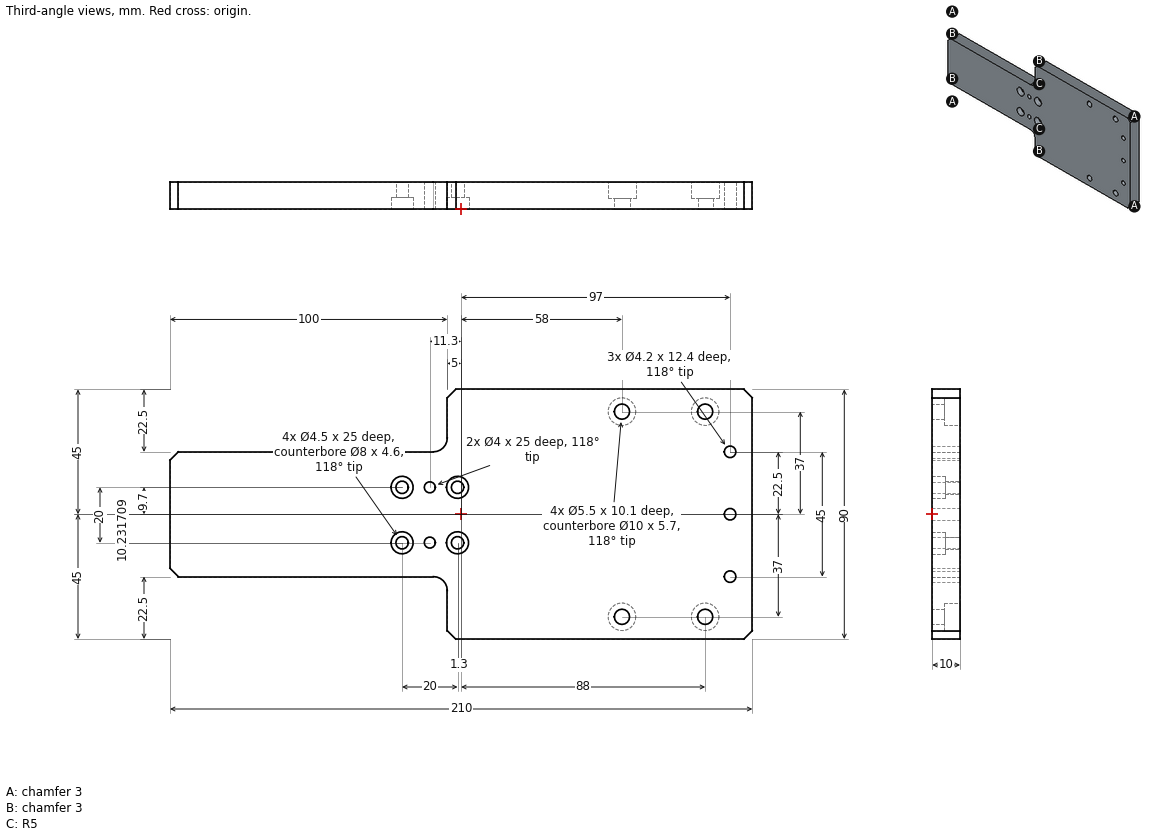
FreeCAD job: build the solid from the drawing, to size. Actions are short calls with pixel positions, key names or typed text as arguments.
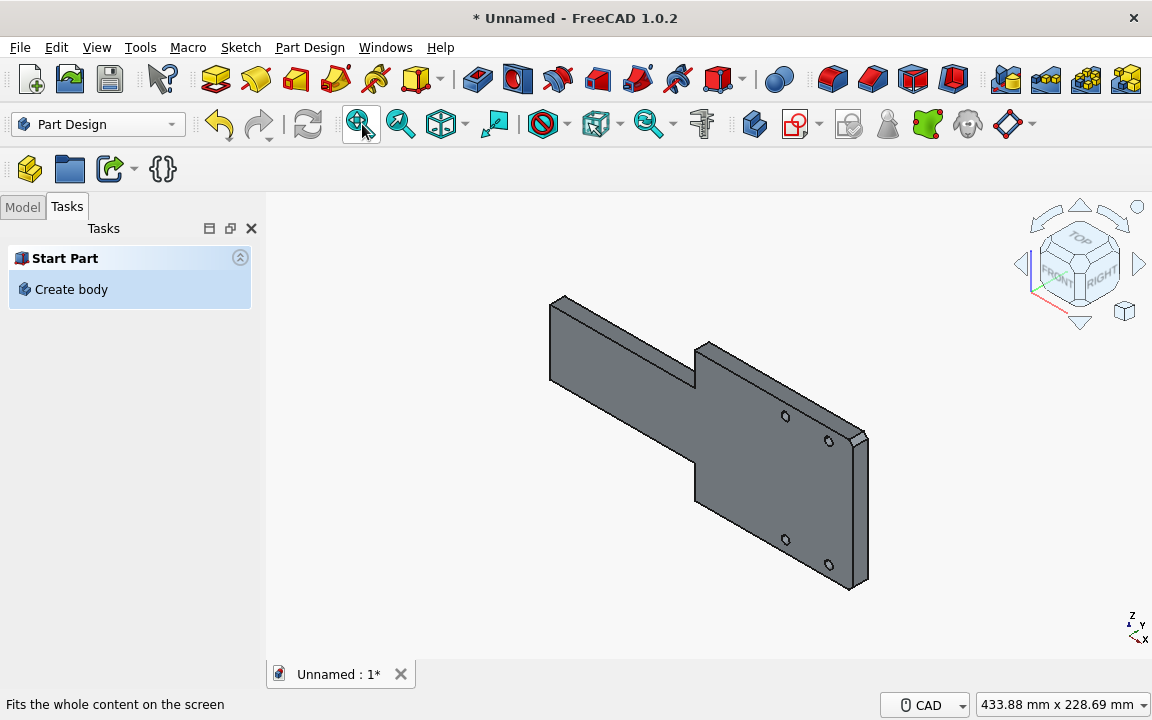
key(2)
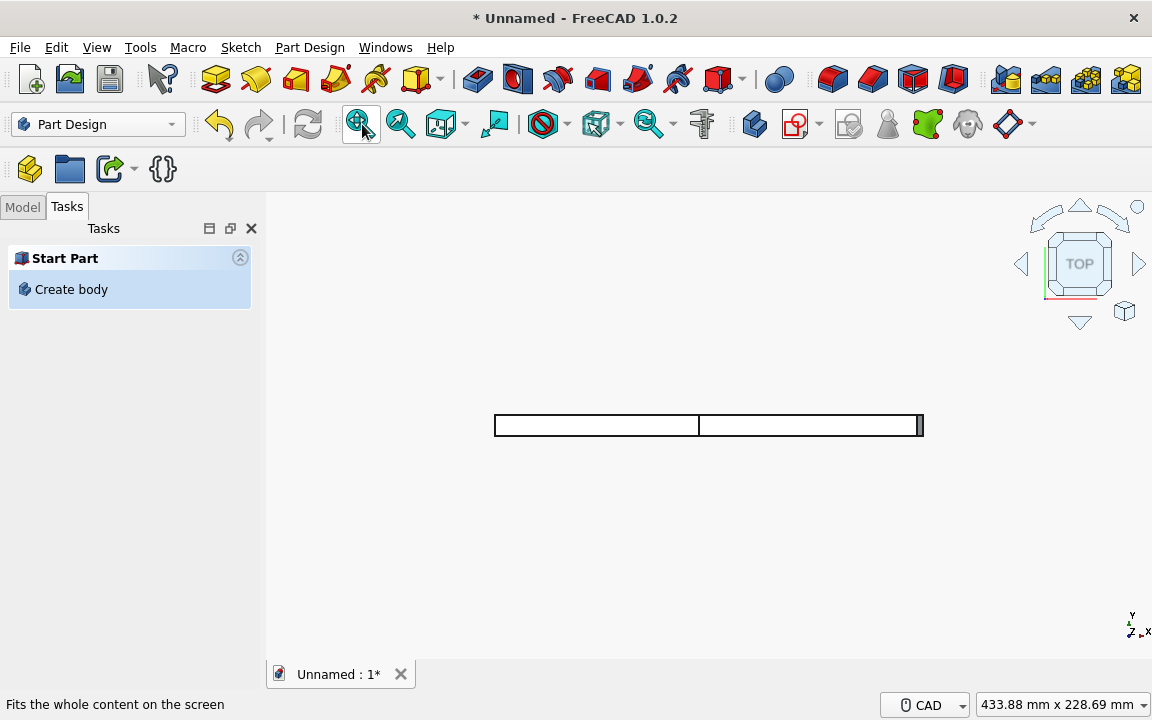
click(495, 424)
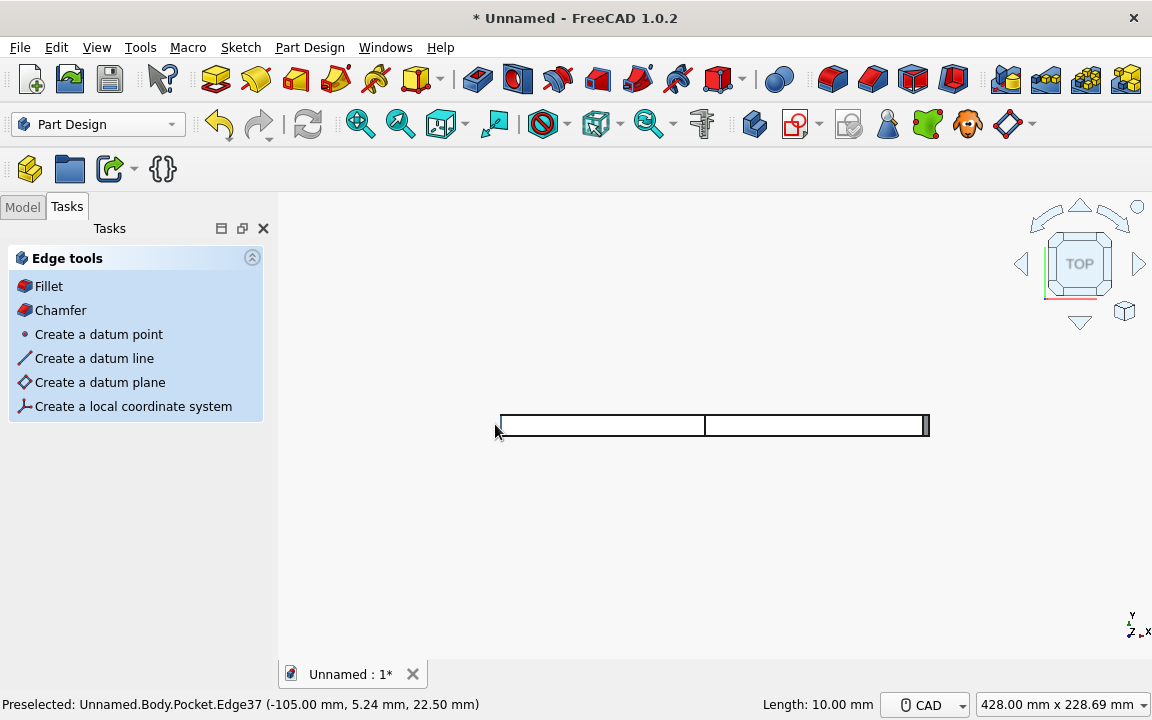
click(705, 424, ctrl)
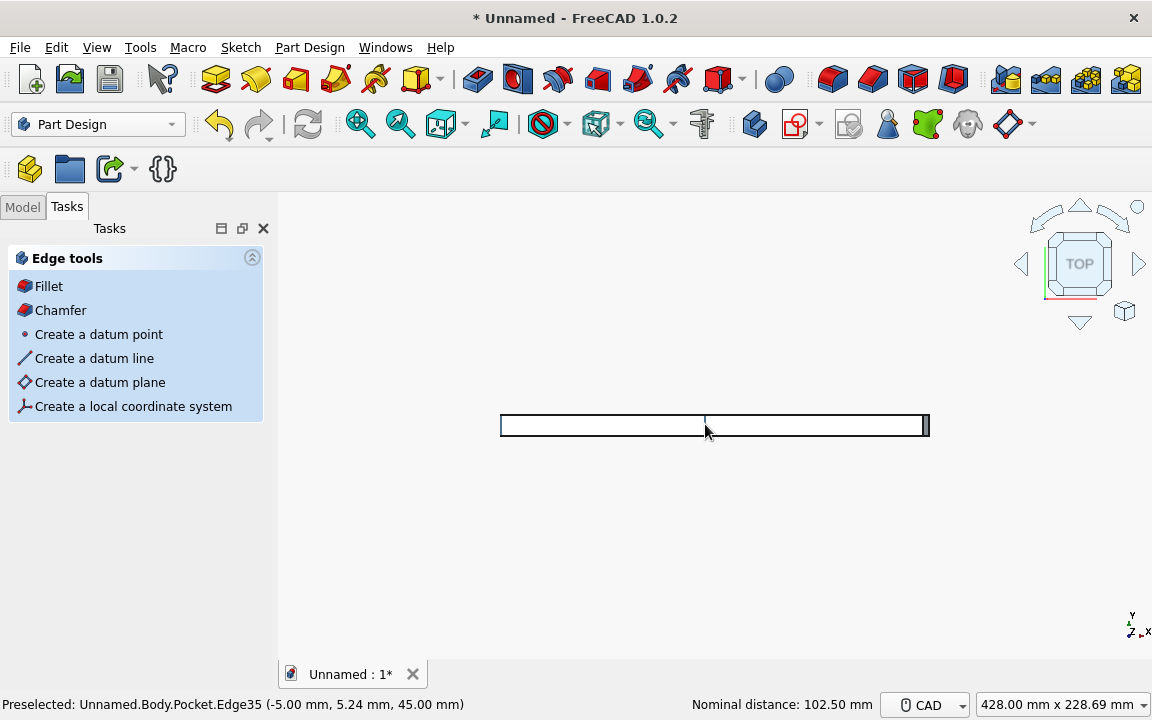
scroll(705, 424, up, 4)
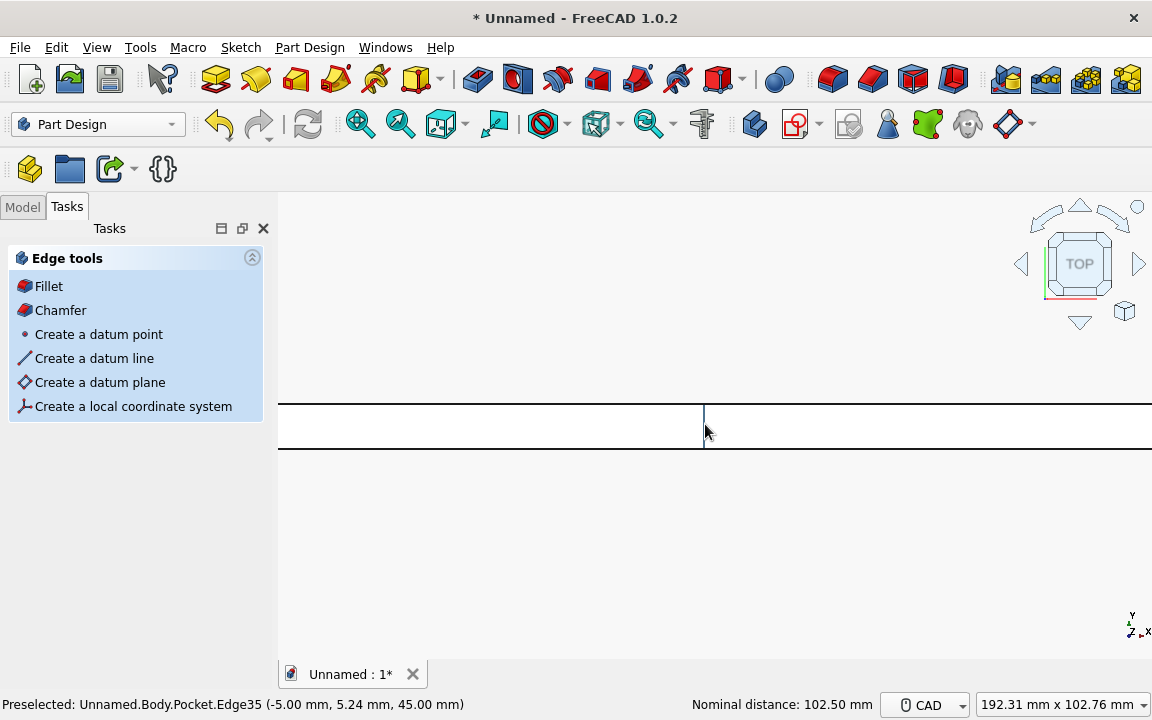
click(362, 124)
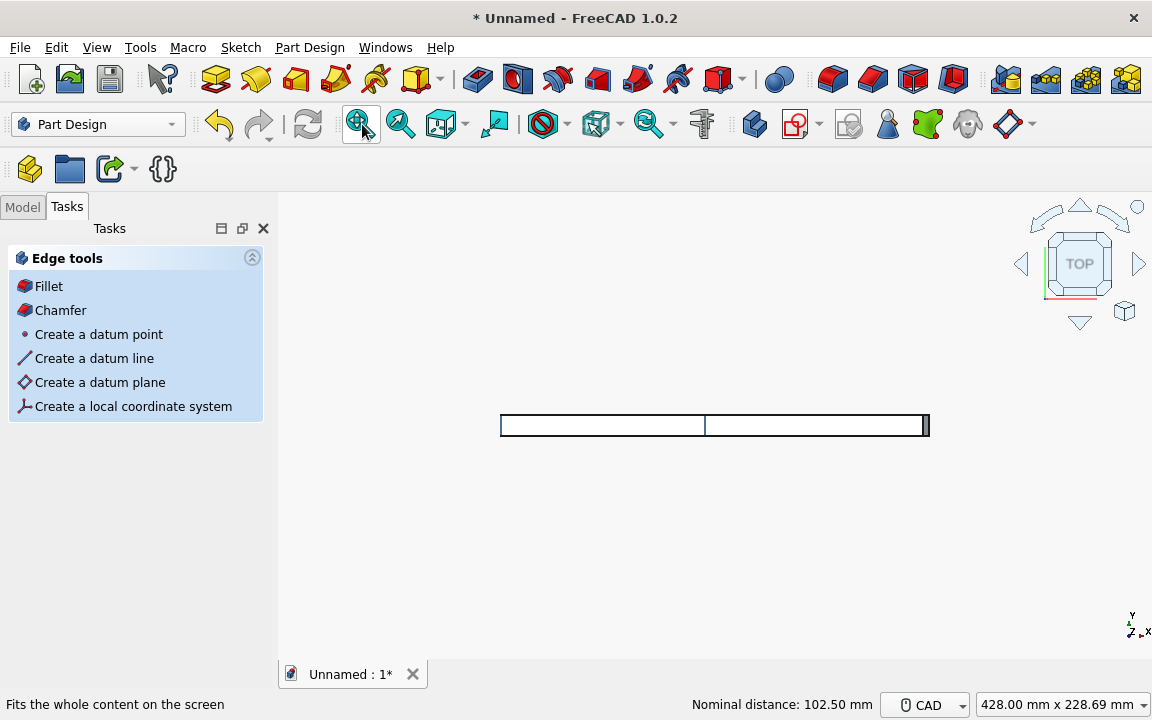
key(1)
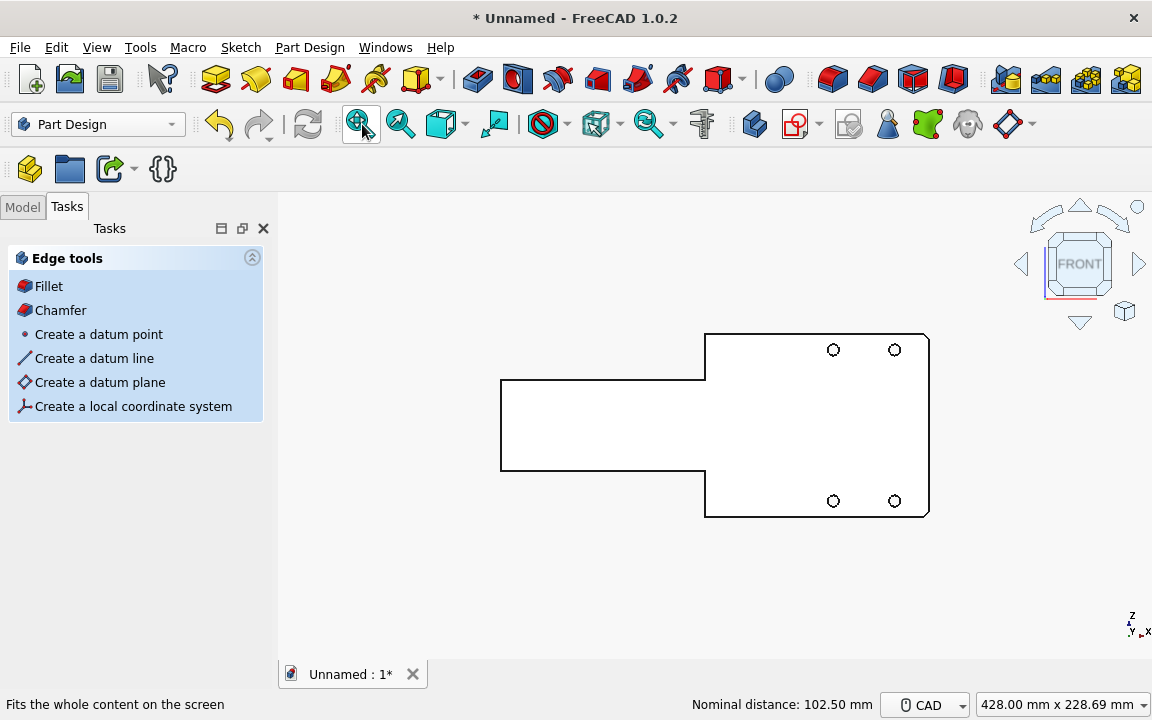
scroll(705, 516, up, 4)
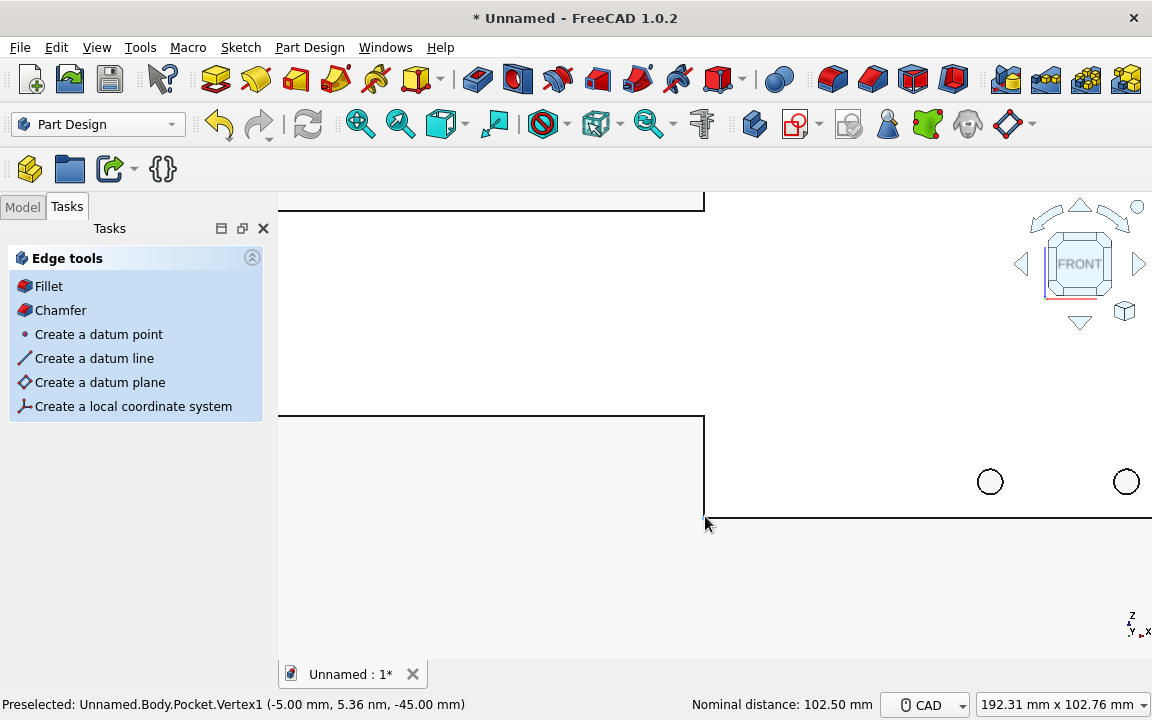
click(362, 124)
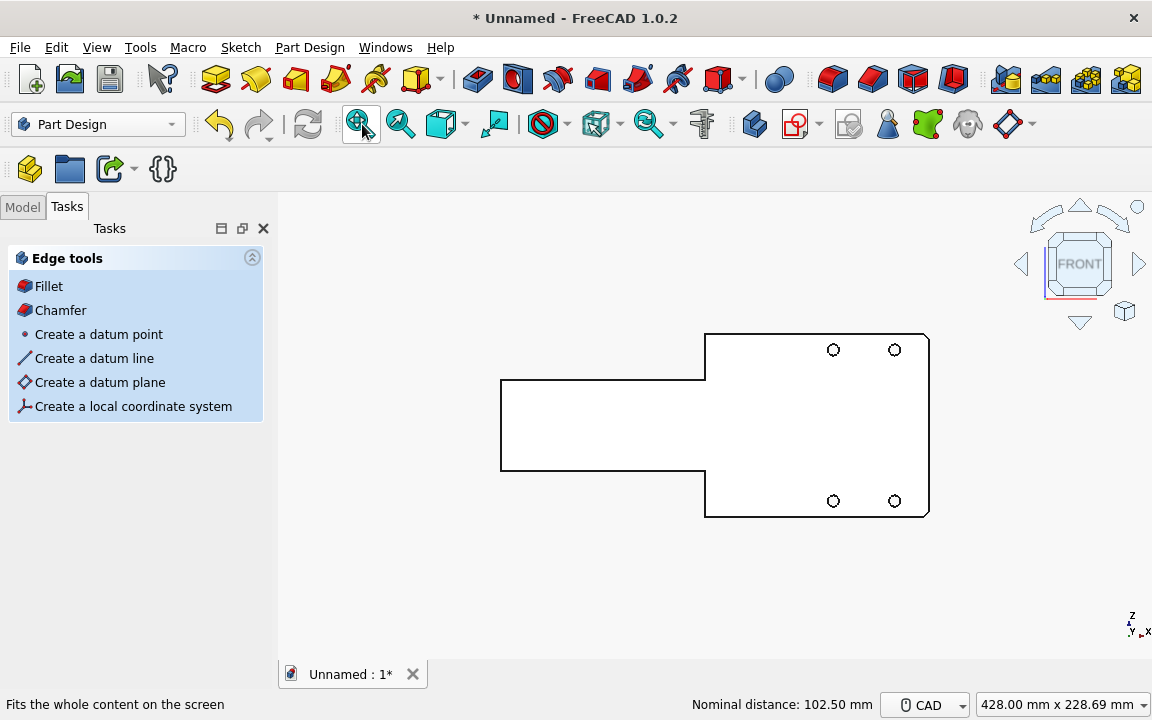
key(3)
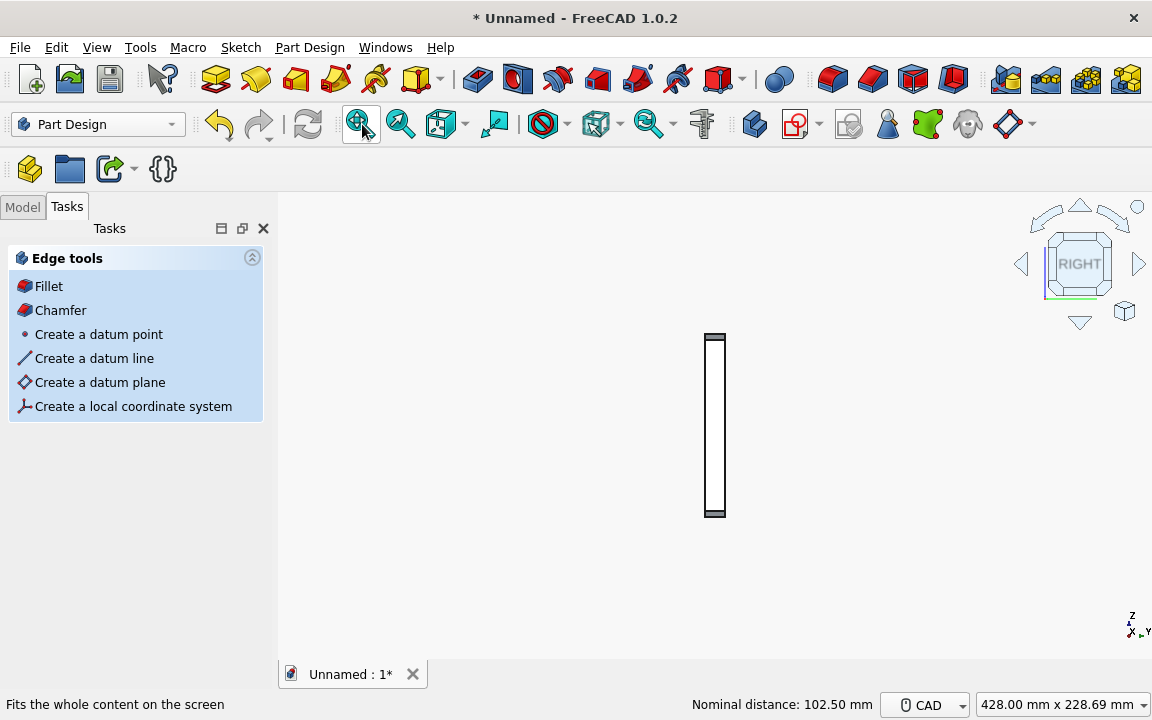
click(362, 124)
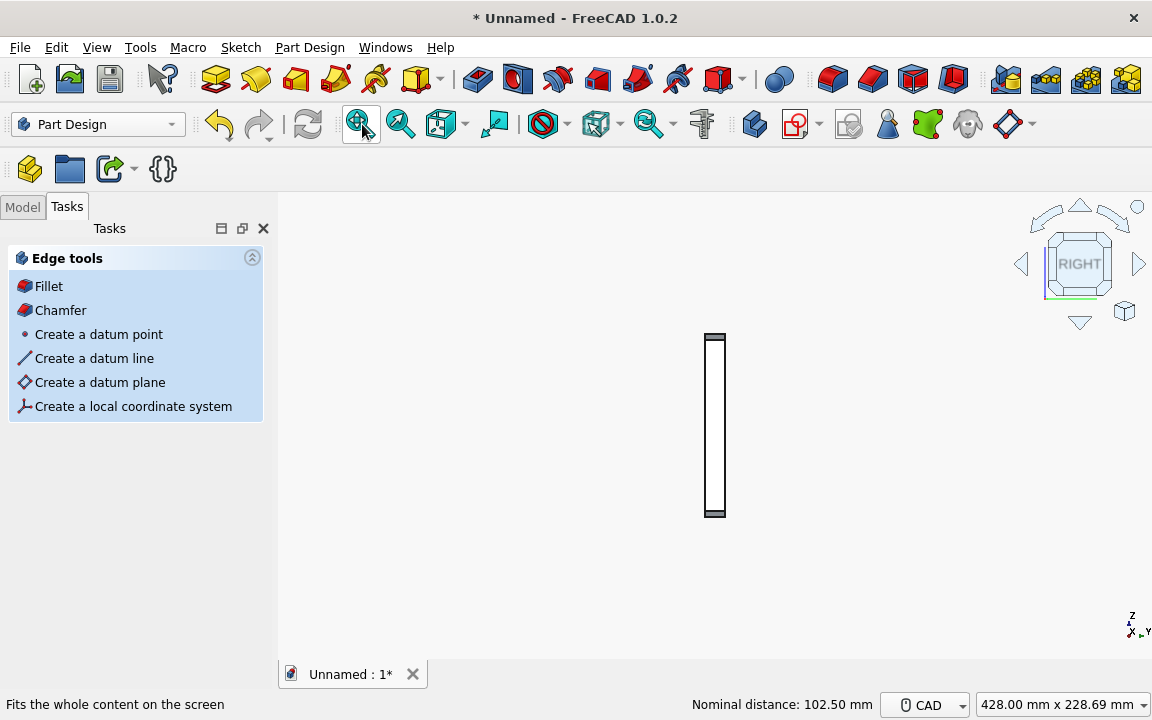
scroll(715, 516, up, 4)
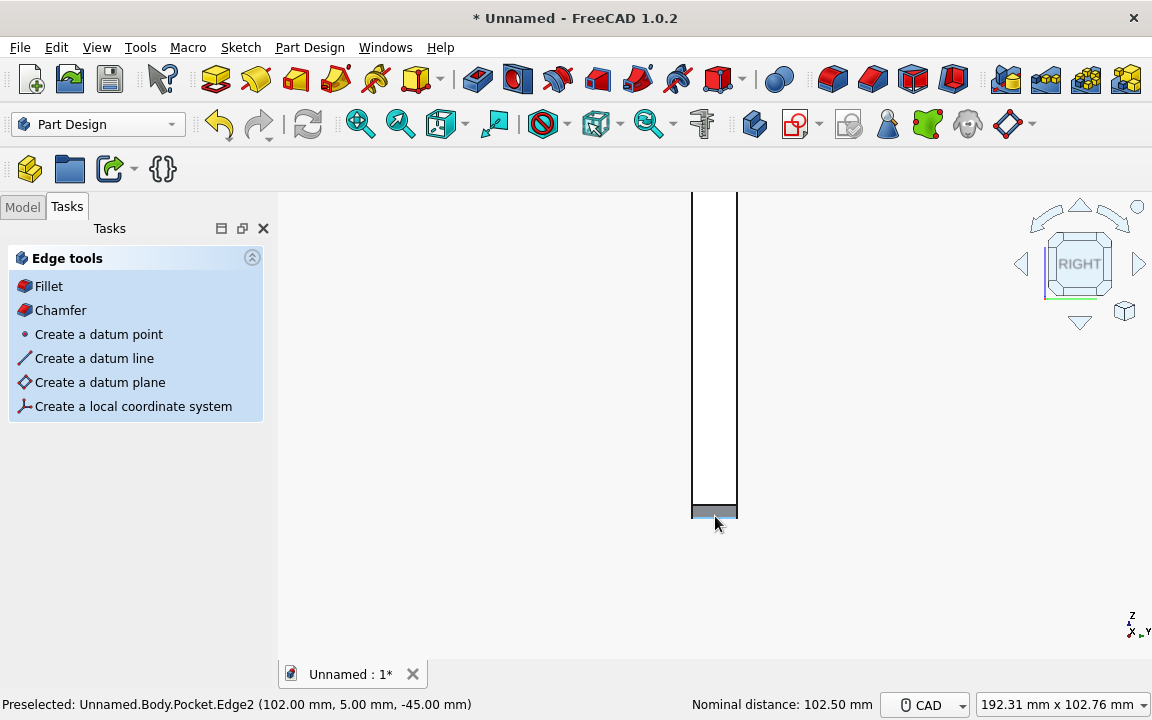
click(362, 124)